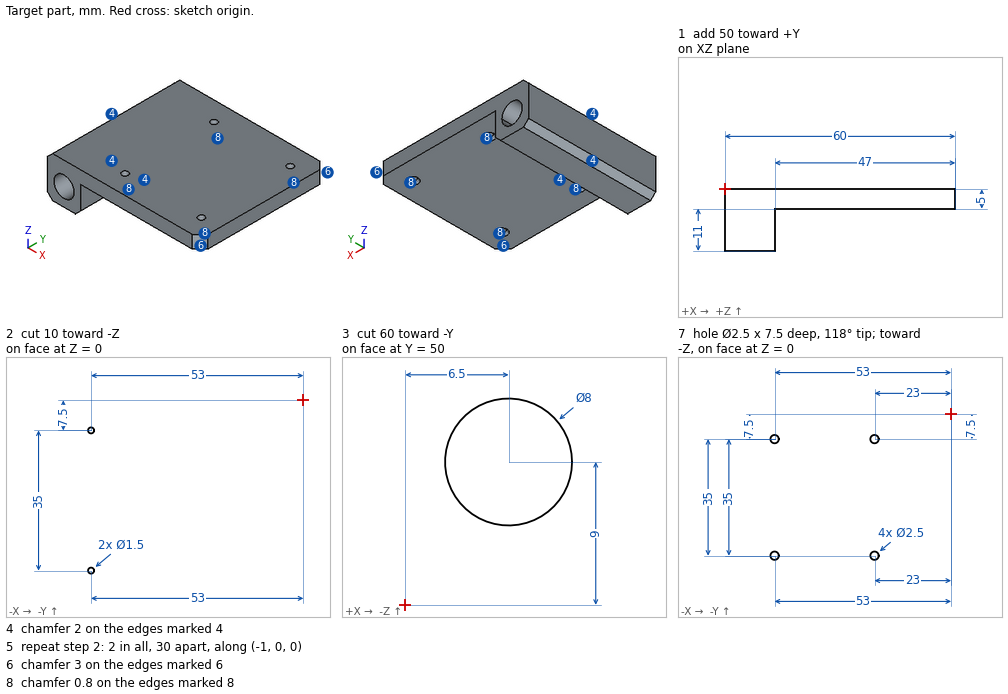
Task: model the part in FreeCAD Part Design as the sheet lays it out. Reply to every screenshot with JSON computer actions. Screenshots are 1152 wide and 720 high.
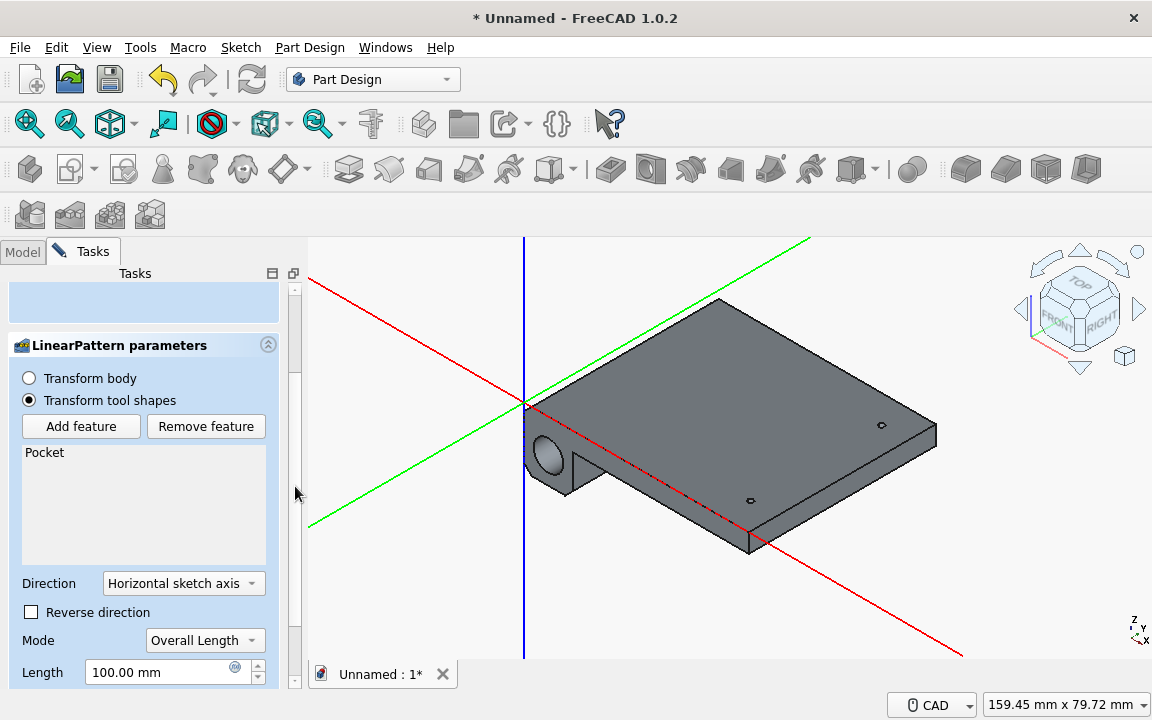
{"action": "left_click", "coordinate": [184, 584]}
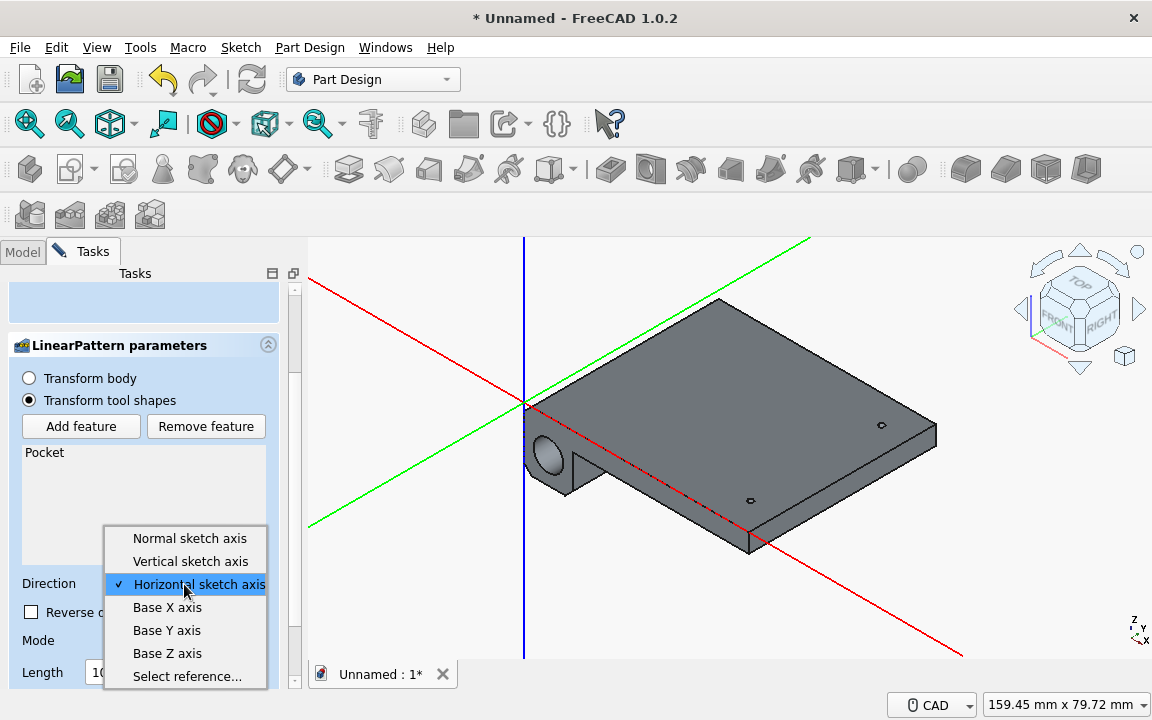
{"action": "left_click", "coordinate": [184, 608]}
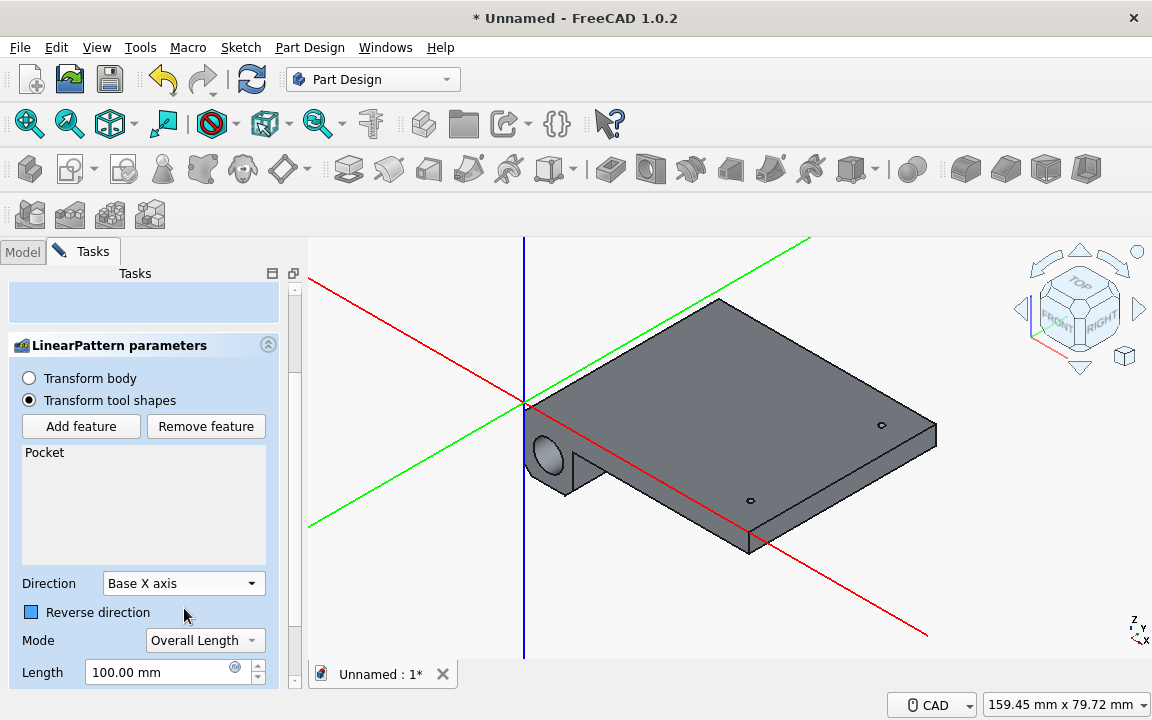
{"action": "left_click", "coordinate": [206, 640]}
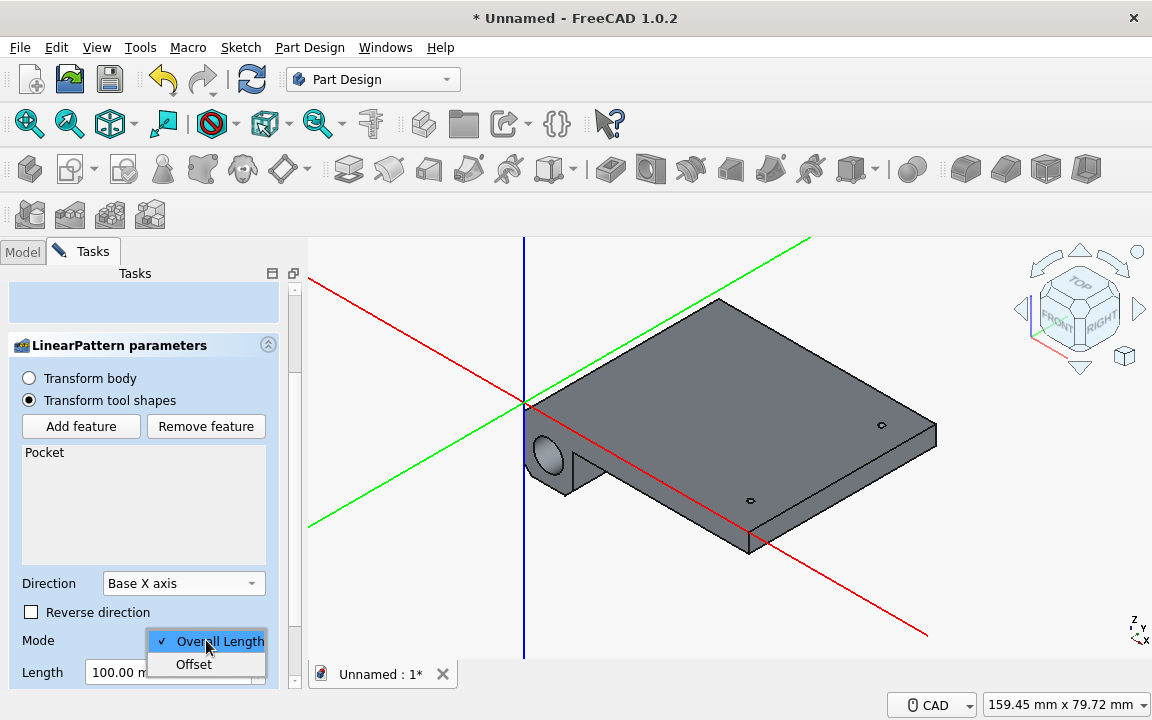
{"action": "left_click", "coordinate": [206, 664]}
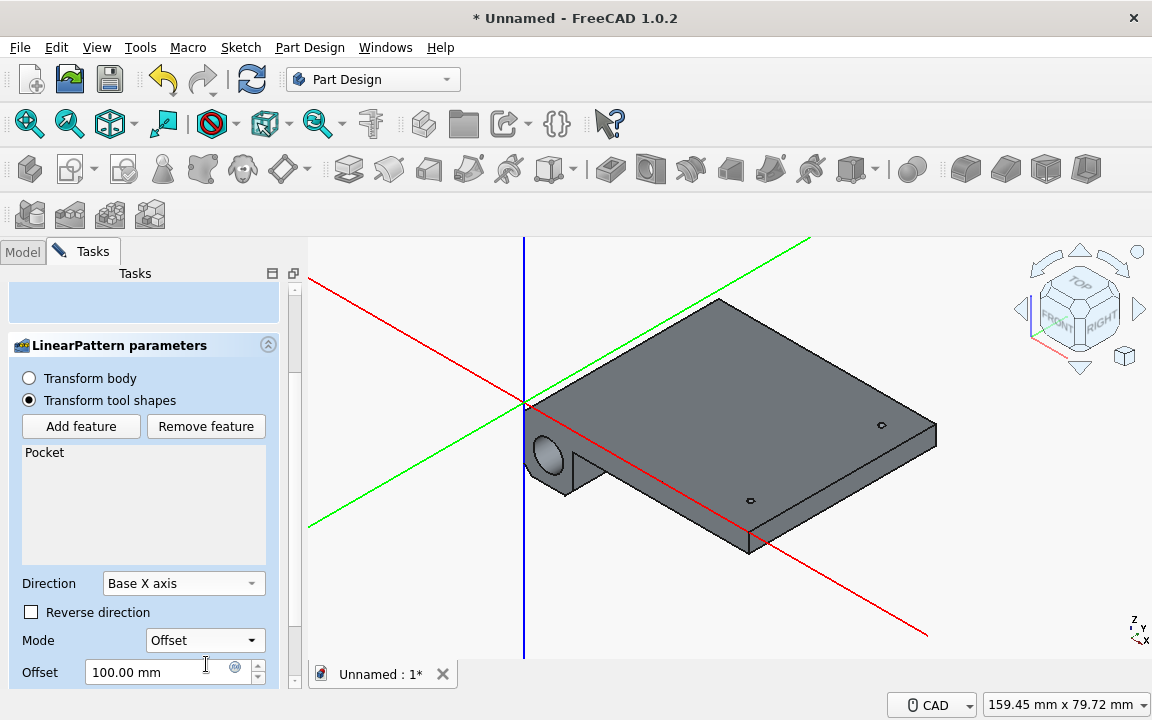
{"action": "triple_click", "coordinate": [168, 672]}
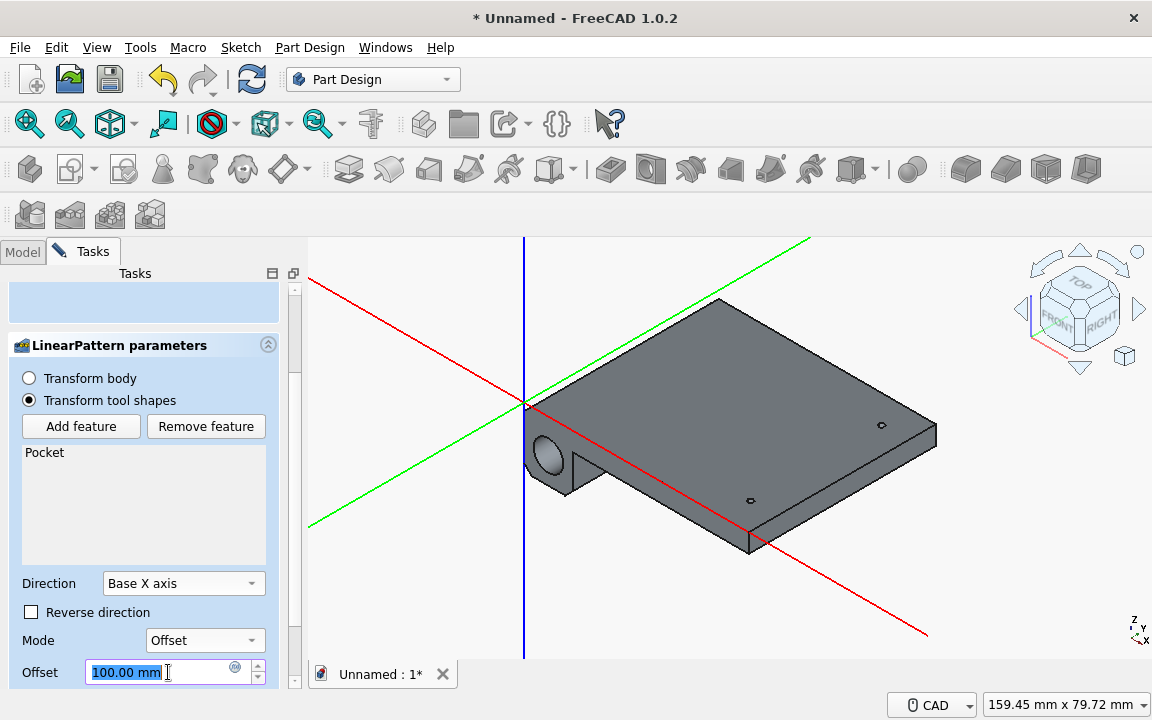
{"action": "type", "text": "30"}
{"action": "key", "text": "Tab"}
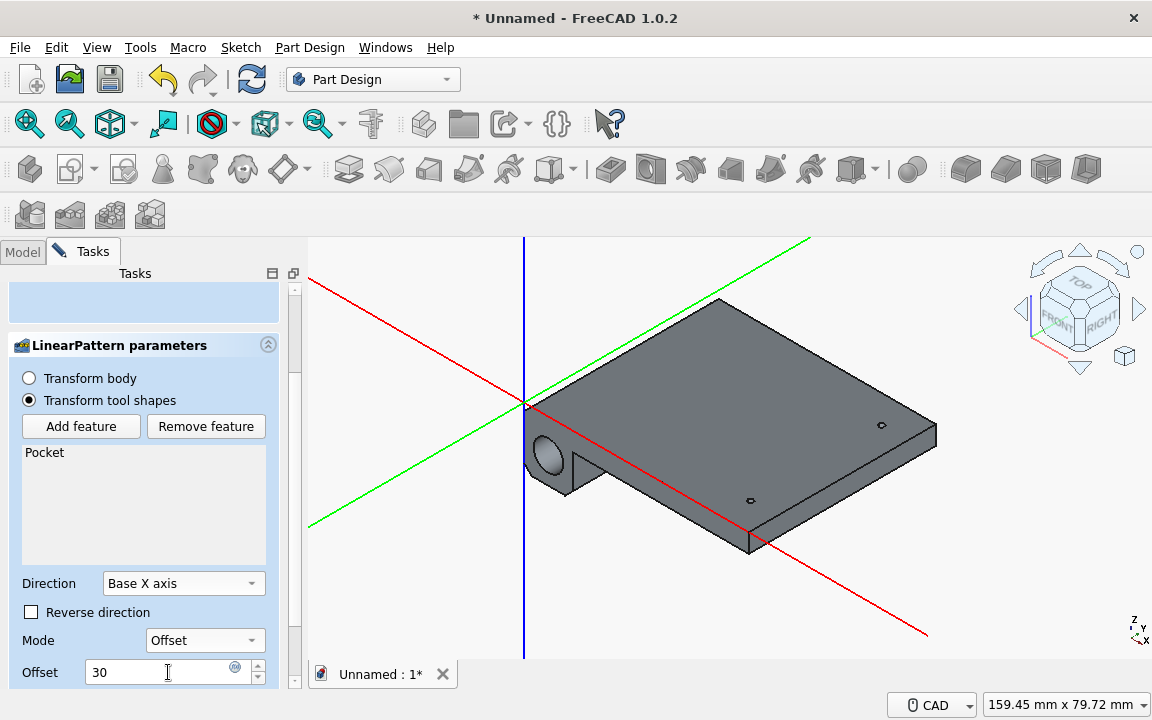
{"action": "scroll", "coordinate": [295, 486], "scroll_direction": "down", "scroll_amount": 2}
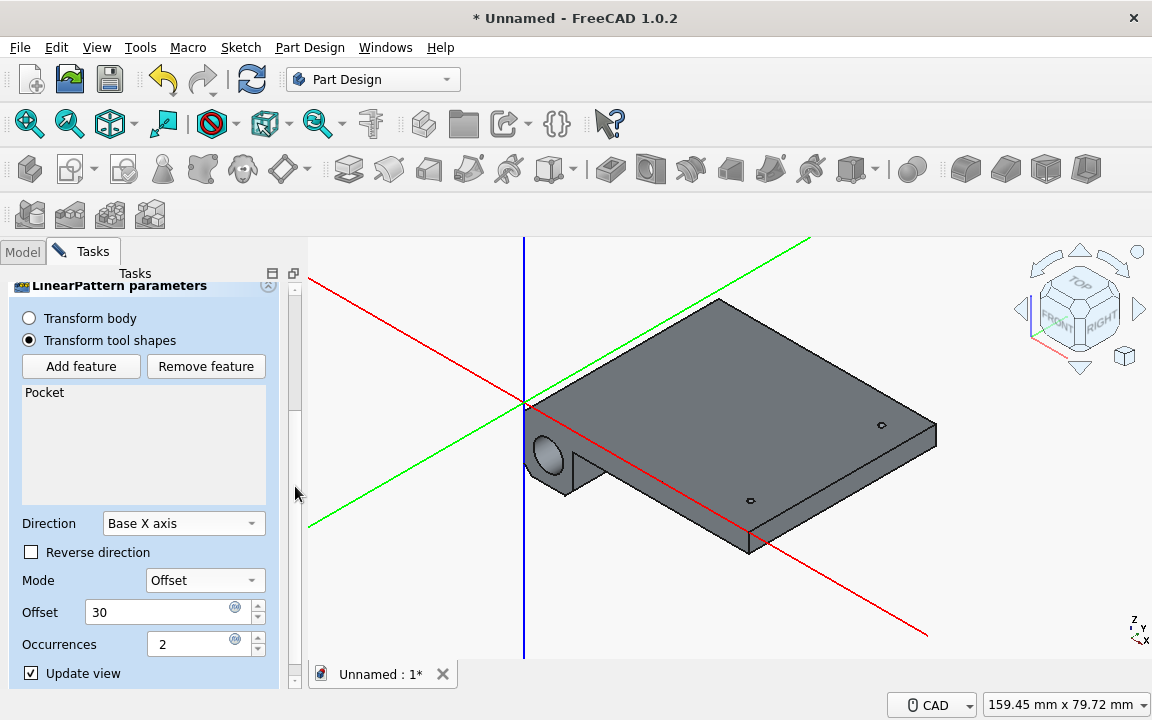
{"action": "triple_click", "coordinate": [198, 628]}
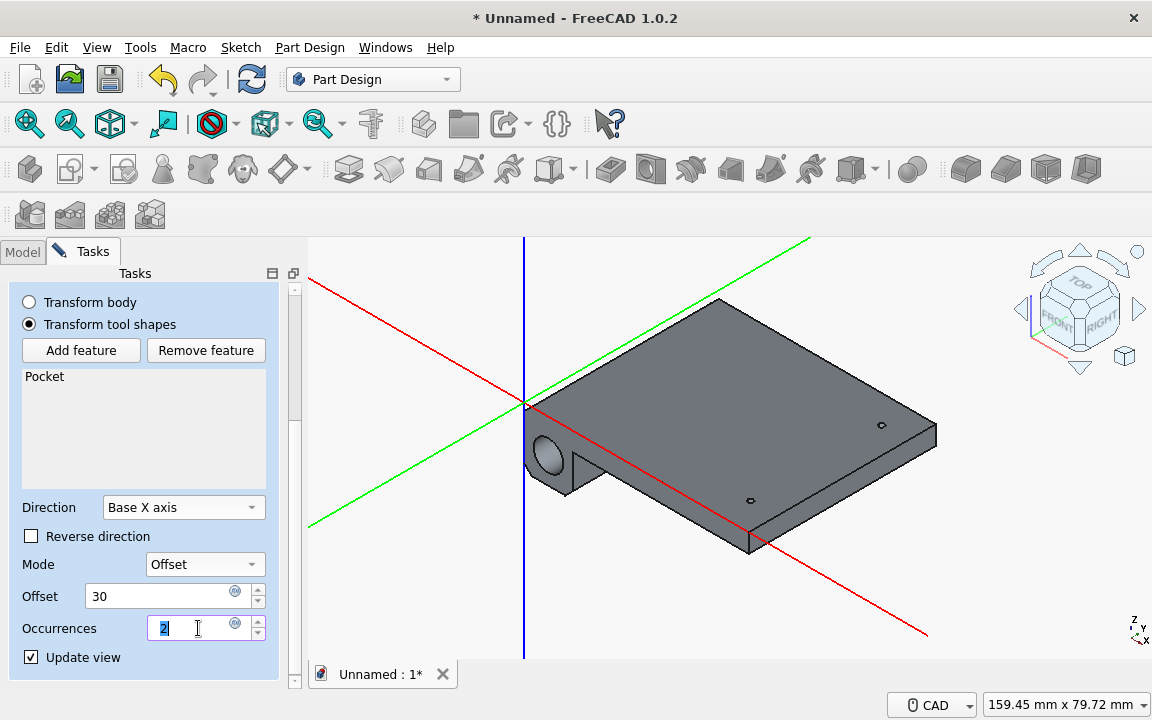
{"action": "type", "text": "2"}
{"action": "key", "text": "Tab"}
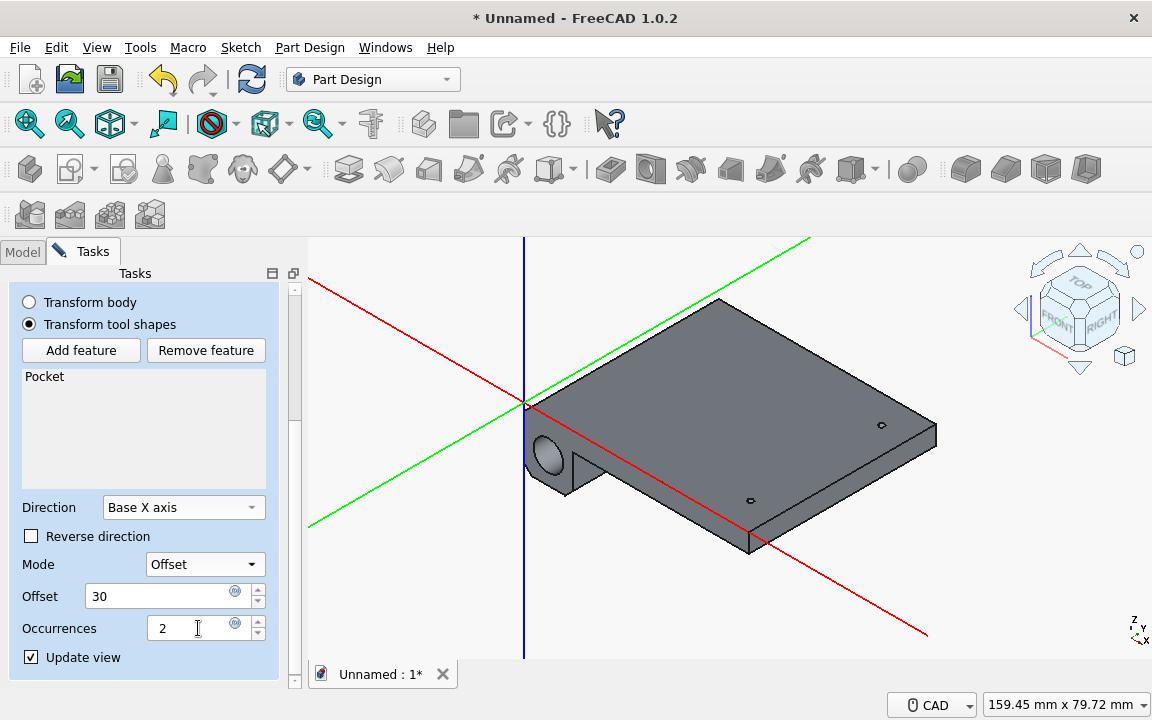
{"action": "left_click", "coordinate": [30, 536]}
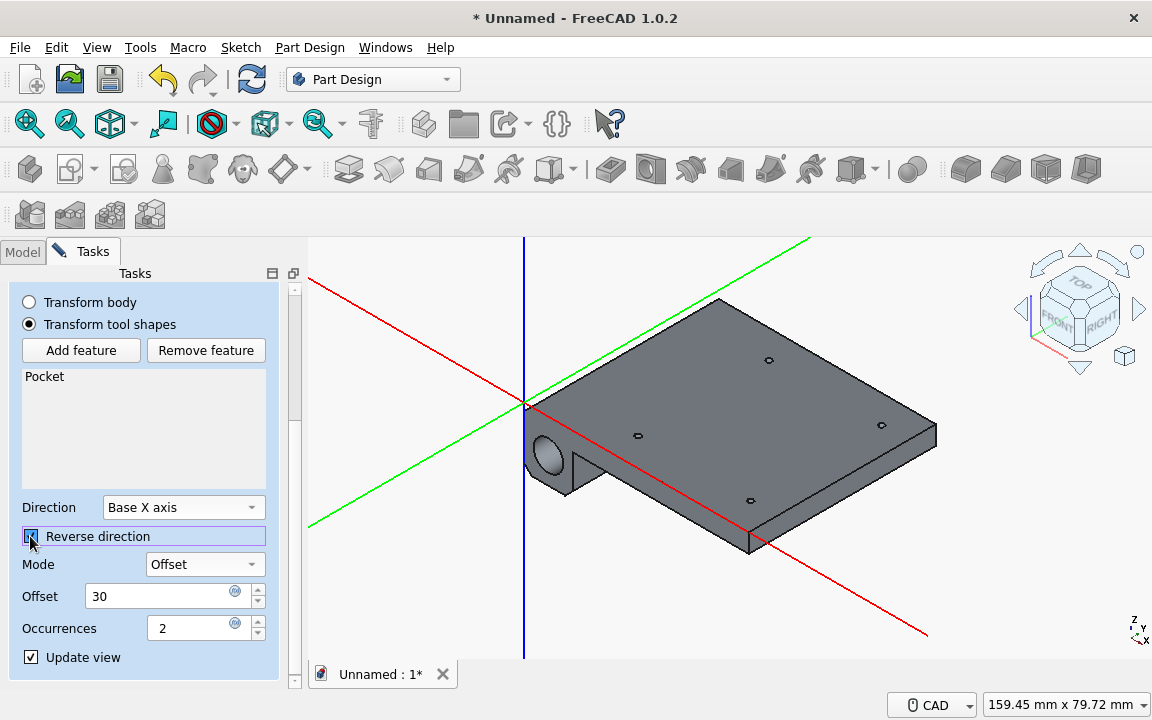
{"action": "scroll", "coordinate": [295, 486], "scroll_direction": "up", "scroll_amount": 5}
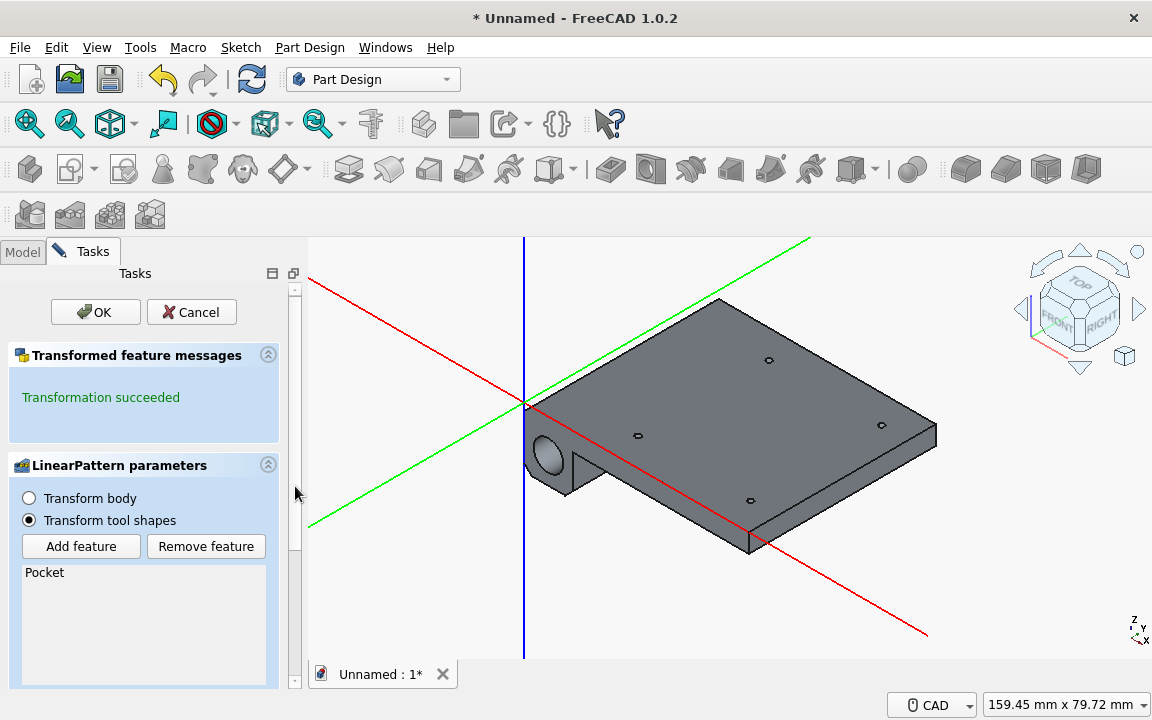
{"action": "left_click", "coordinate": [96, 312]}